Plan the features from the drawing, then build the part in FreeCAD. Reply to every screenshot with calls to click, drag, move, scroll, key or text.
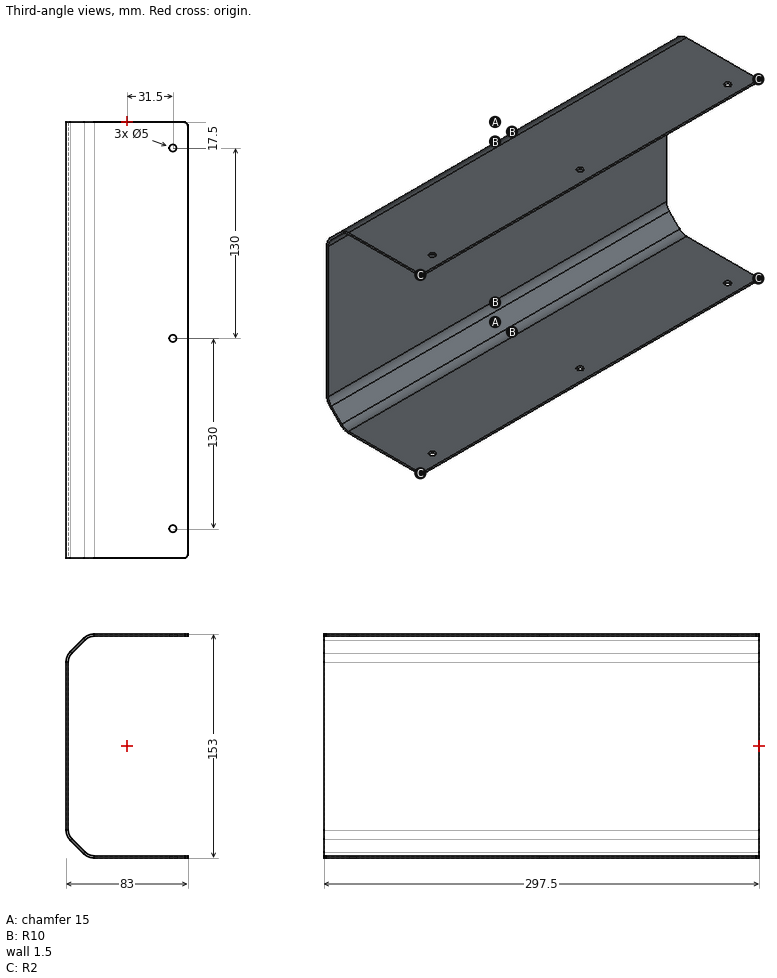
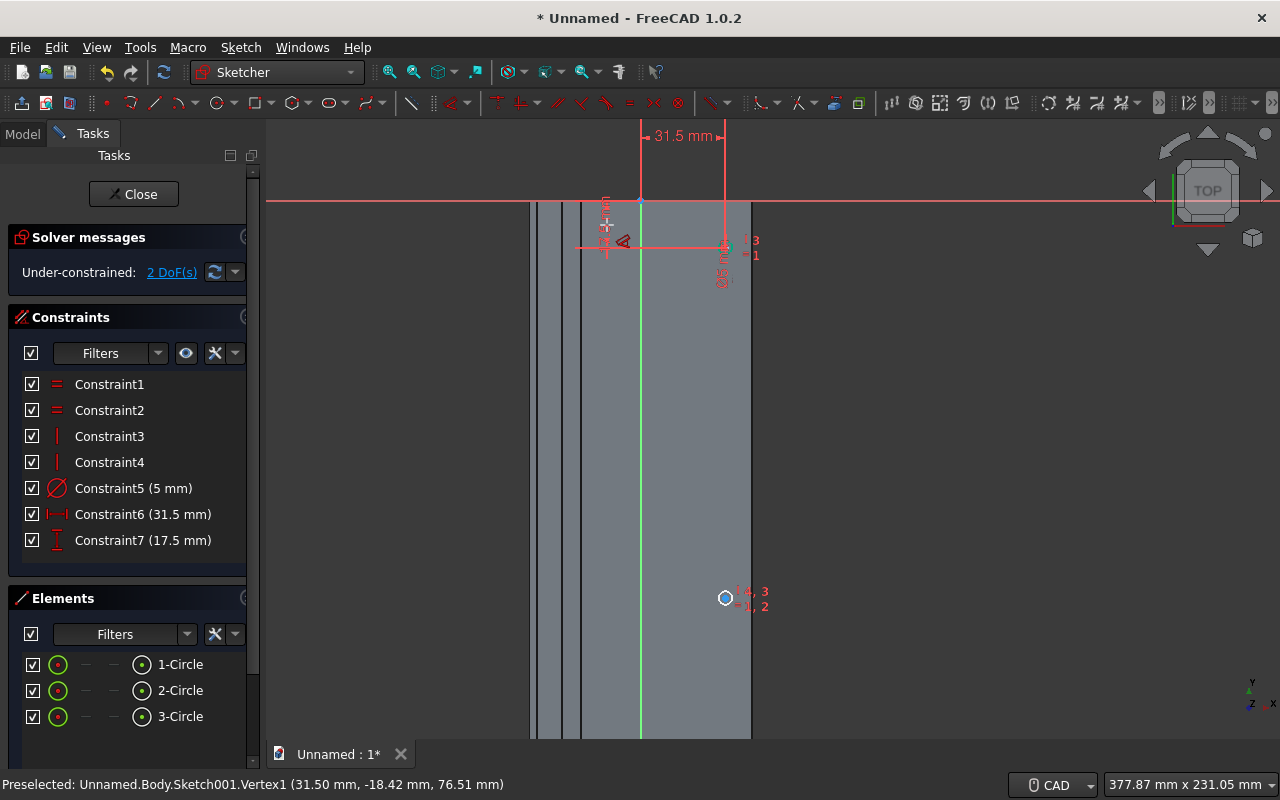
click(725, 248)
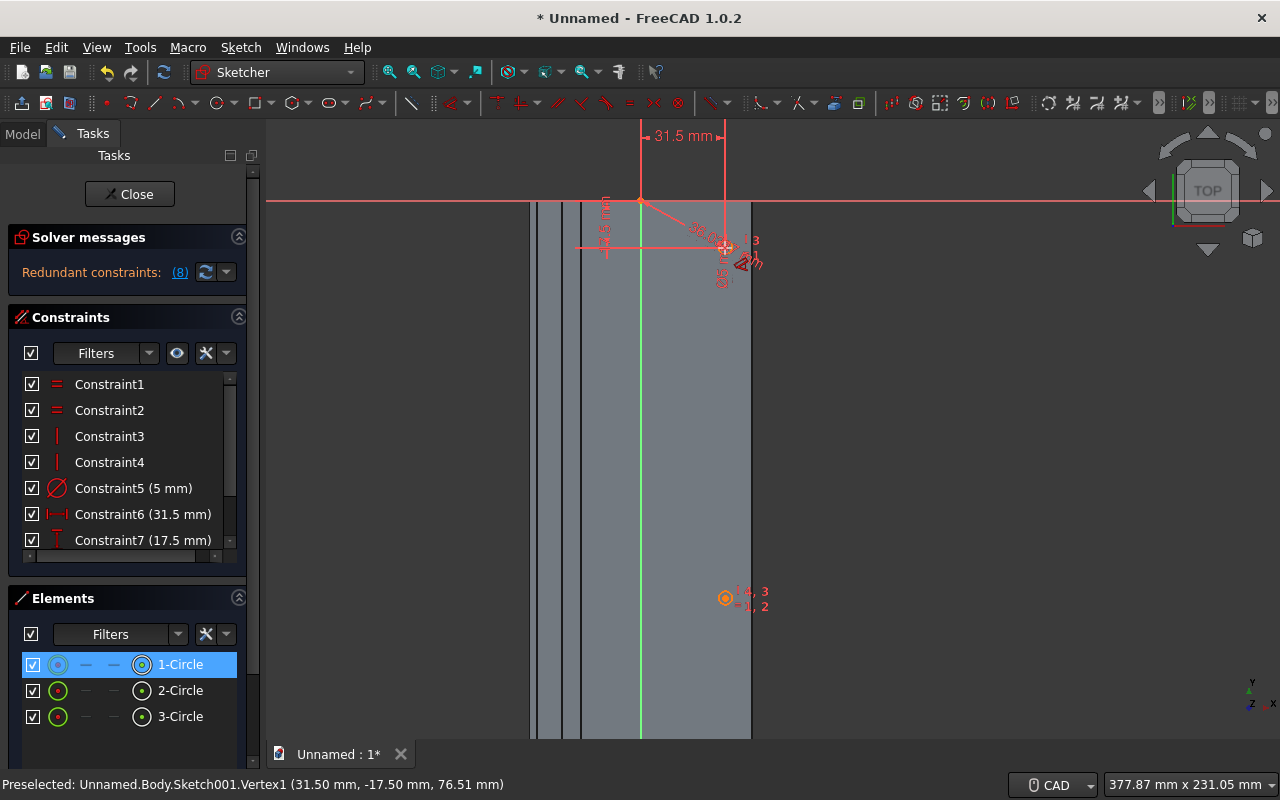
click(725, 598)
click(759, 423)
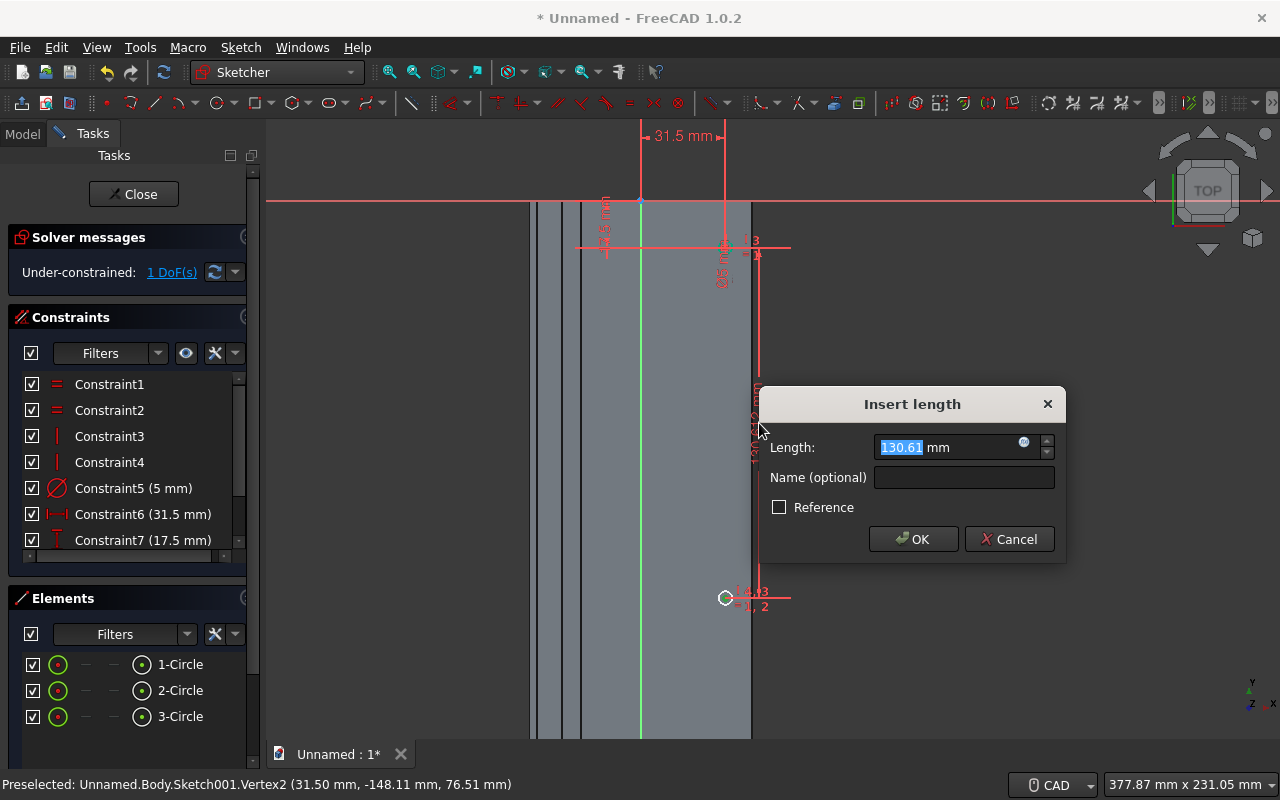
text(130)
key(Return)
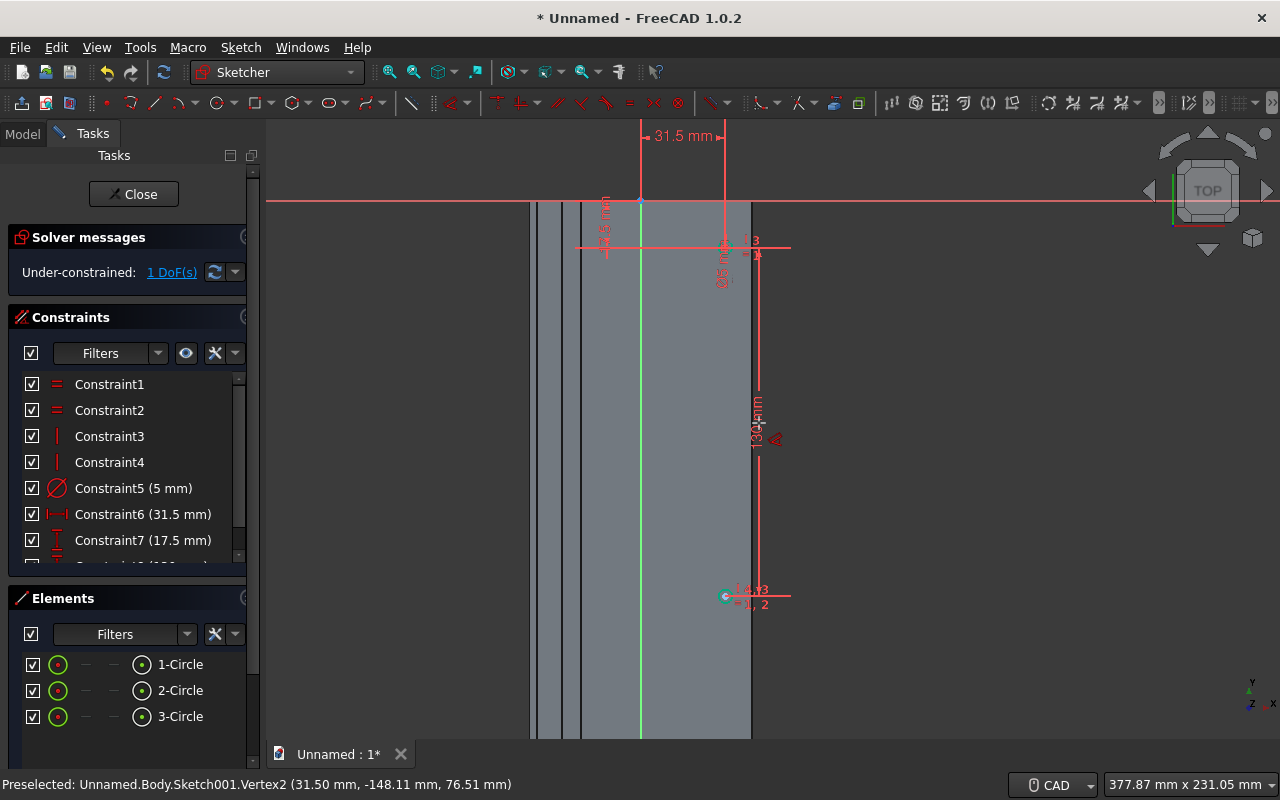
click(725, 596)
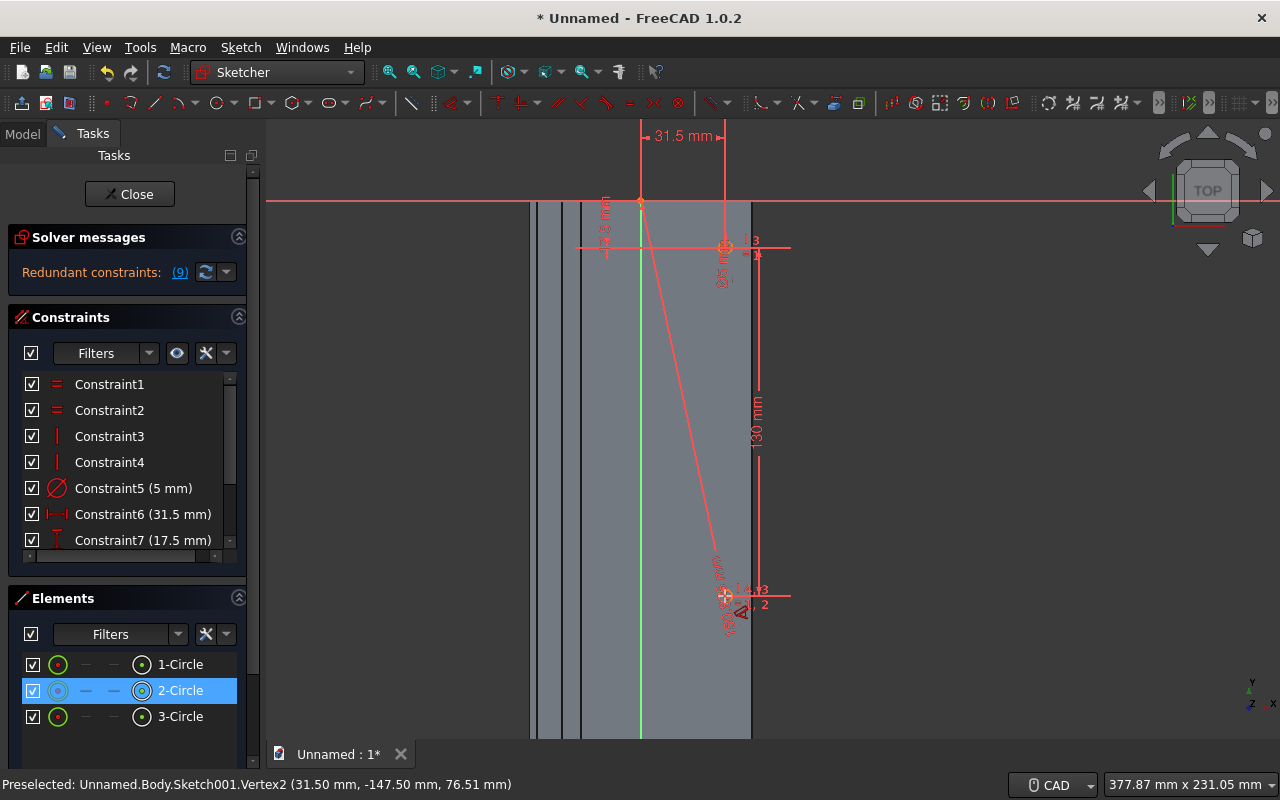
scroll(726, 250, down, 3)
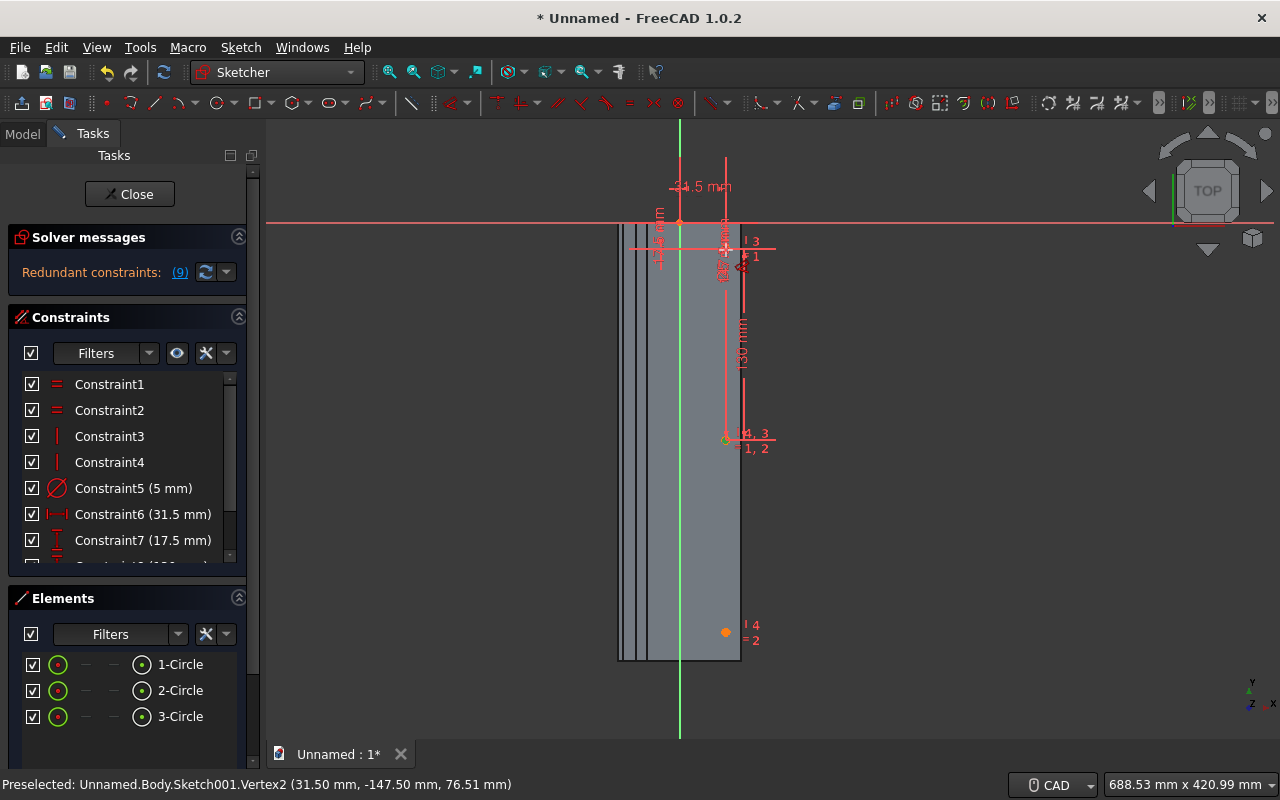
click(726, 632)
click(760, 536)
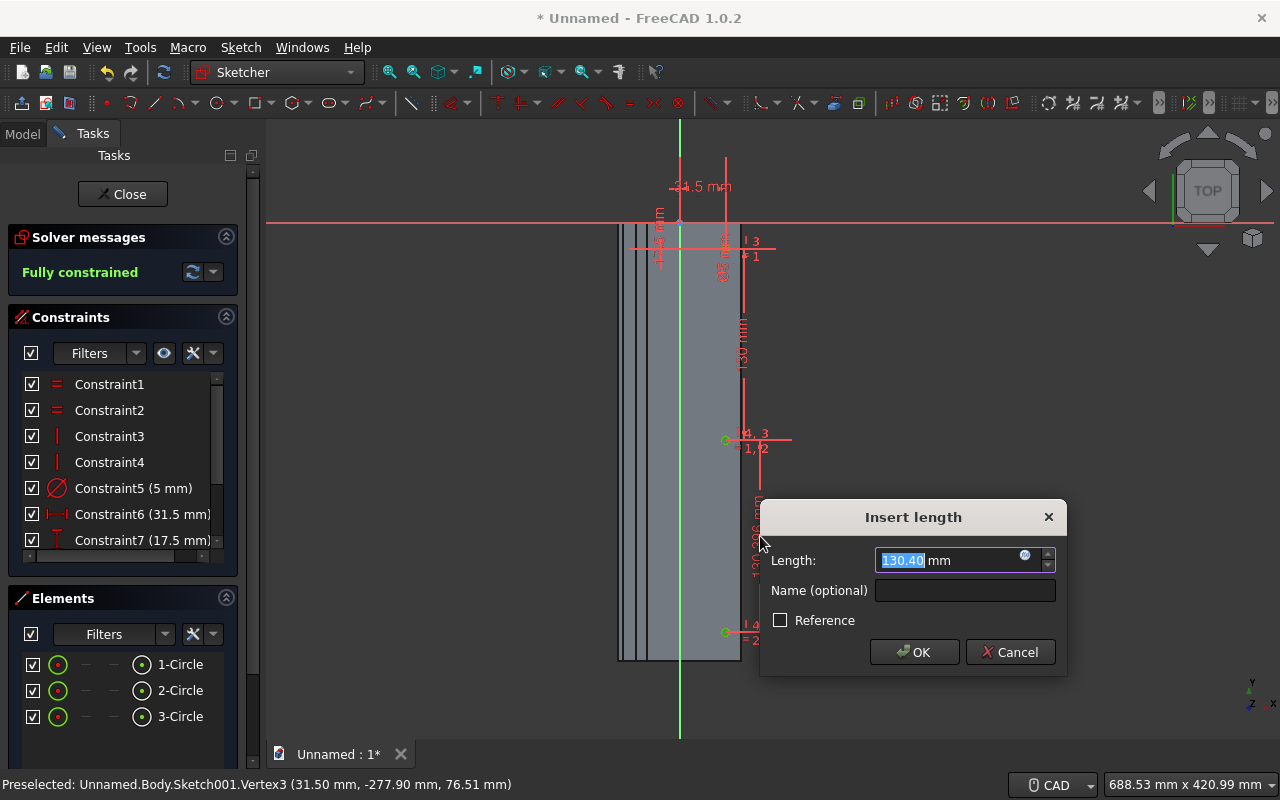
text(130)
key(Return)
key(Escape)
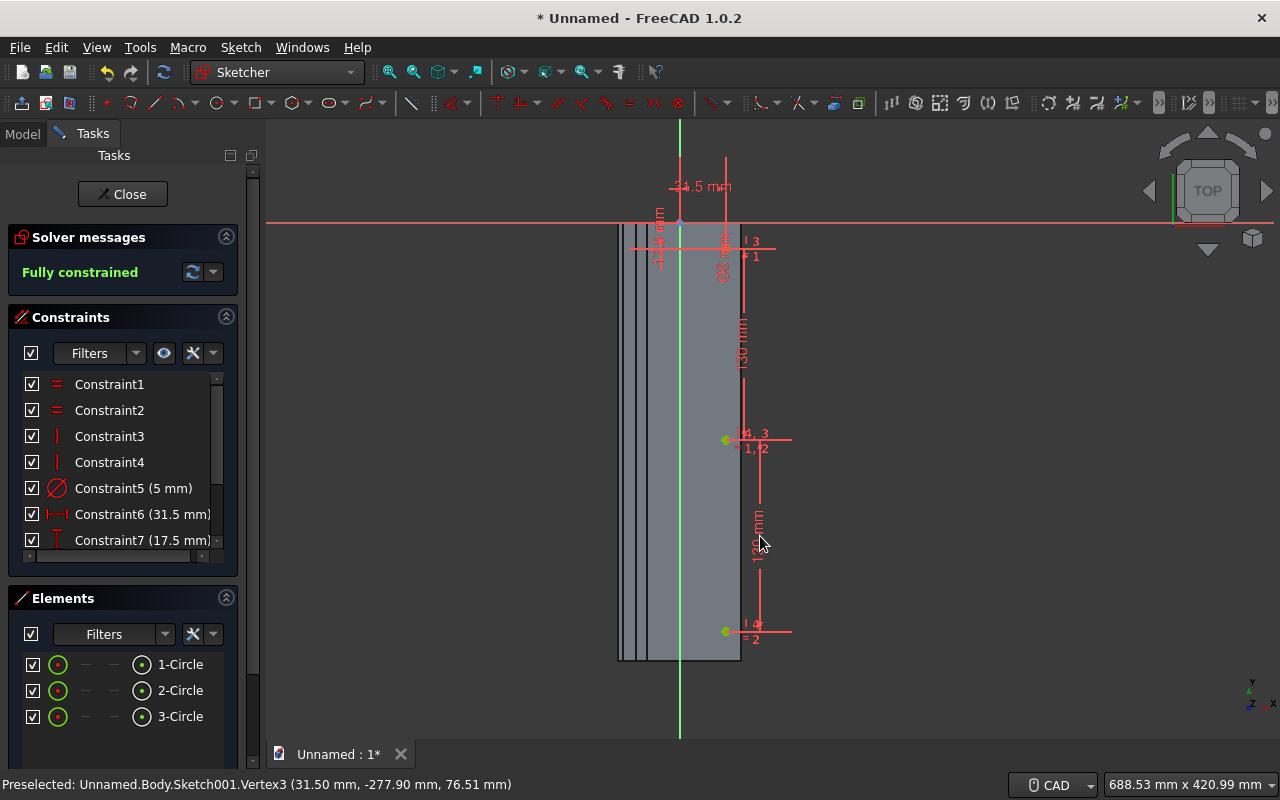
click(123, 194)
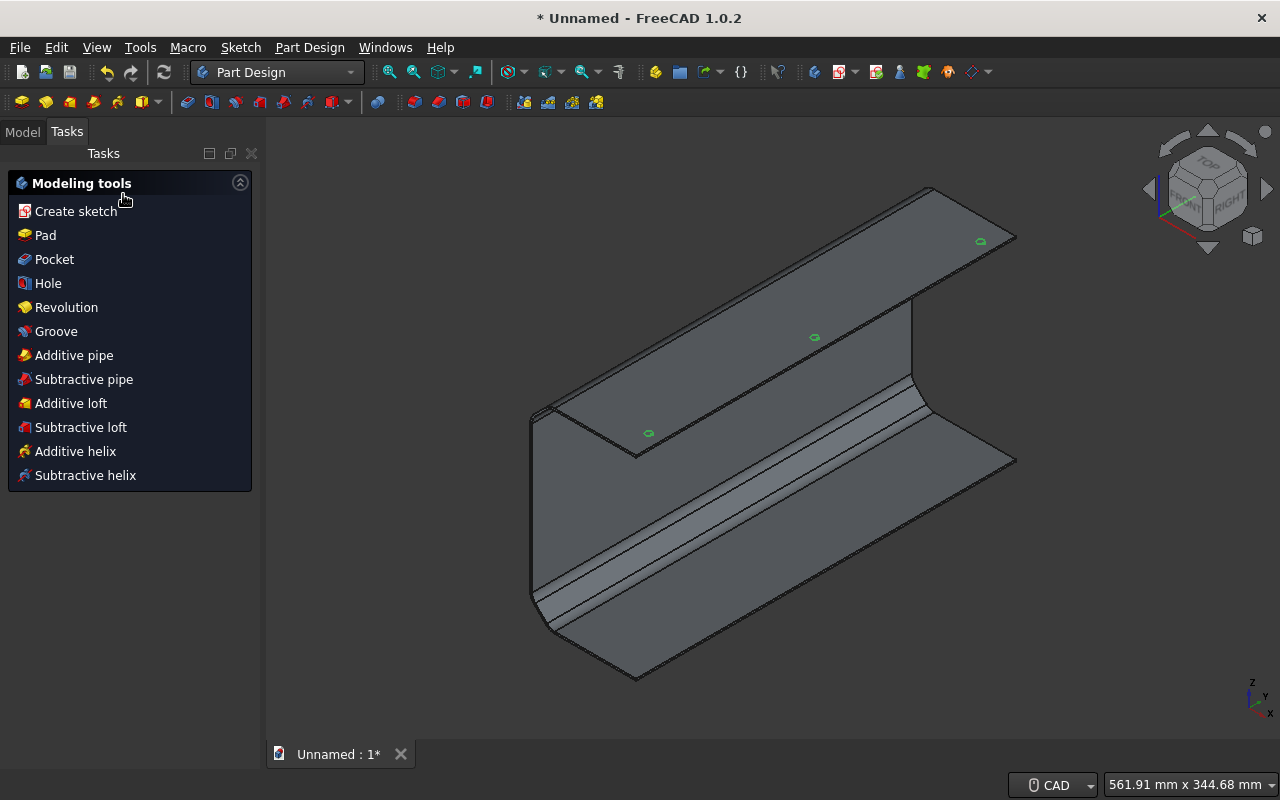
click(188, 102)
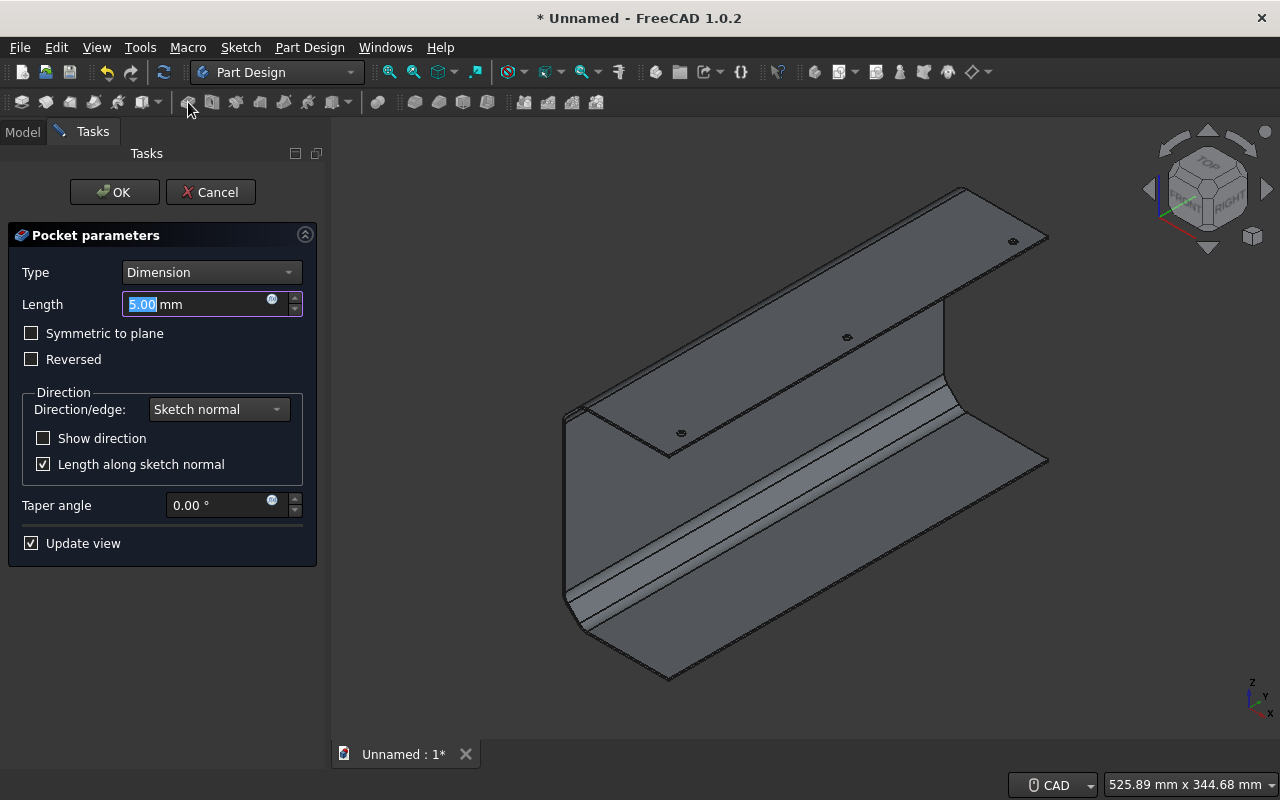
click(212, 272)